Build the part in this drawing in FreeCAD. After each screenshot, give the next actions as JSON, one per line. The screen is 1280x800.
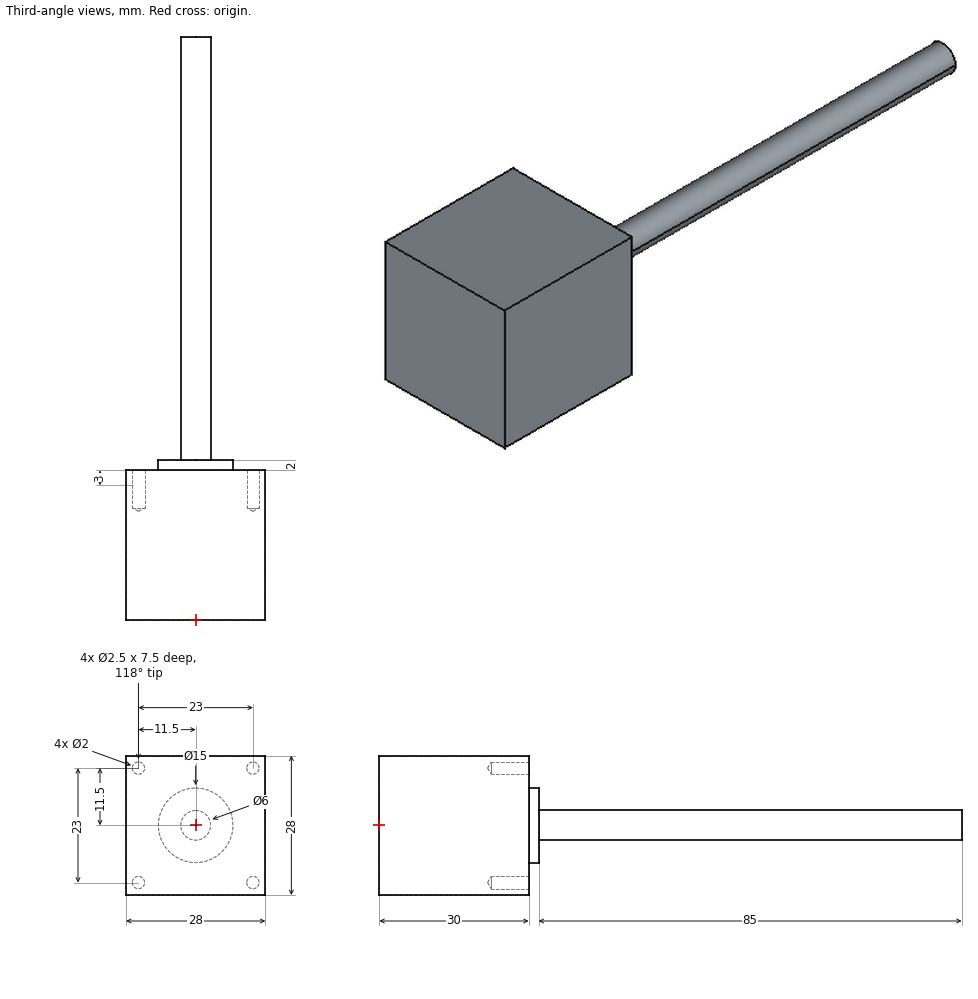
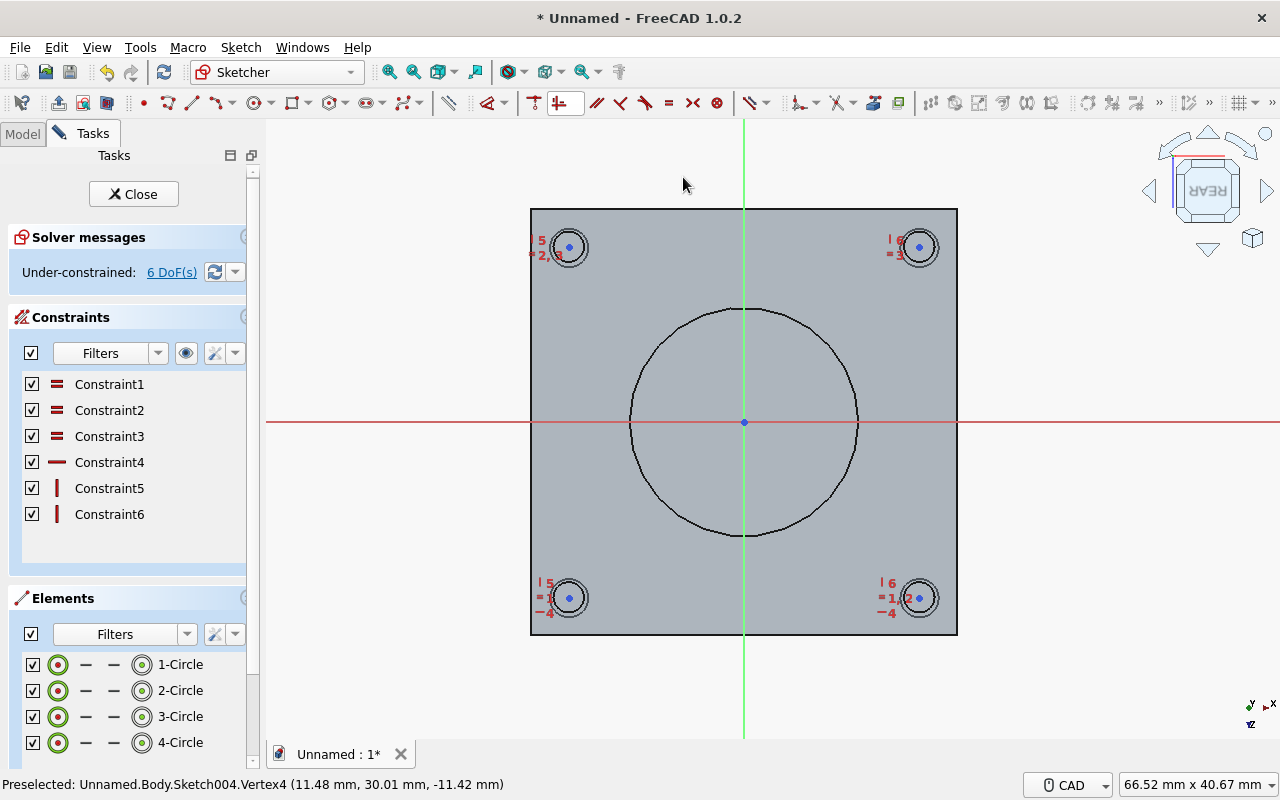
{"action": "left_click", "coordinate": [569, 248]}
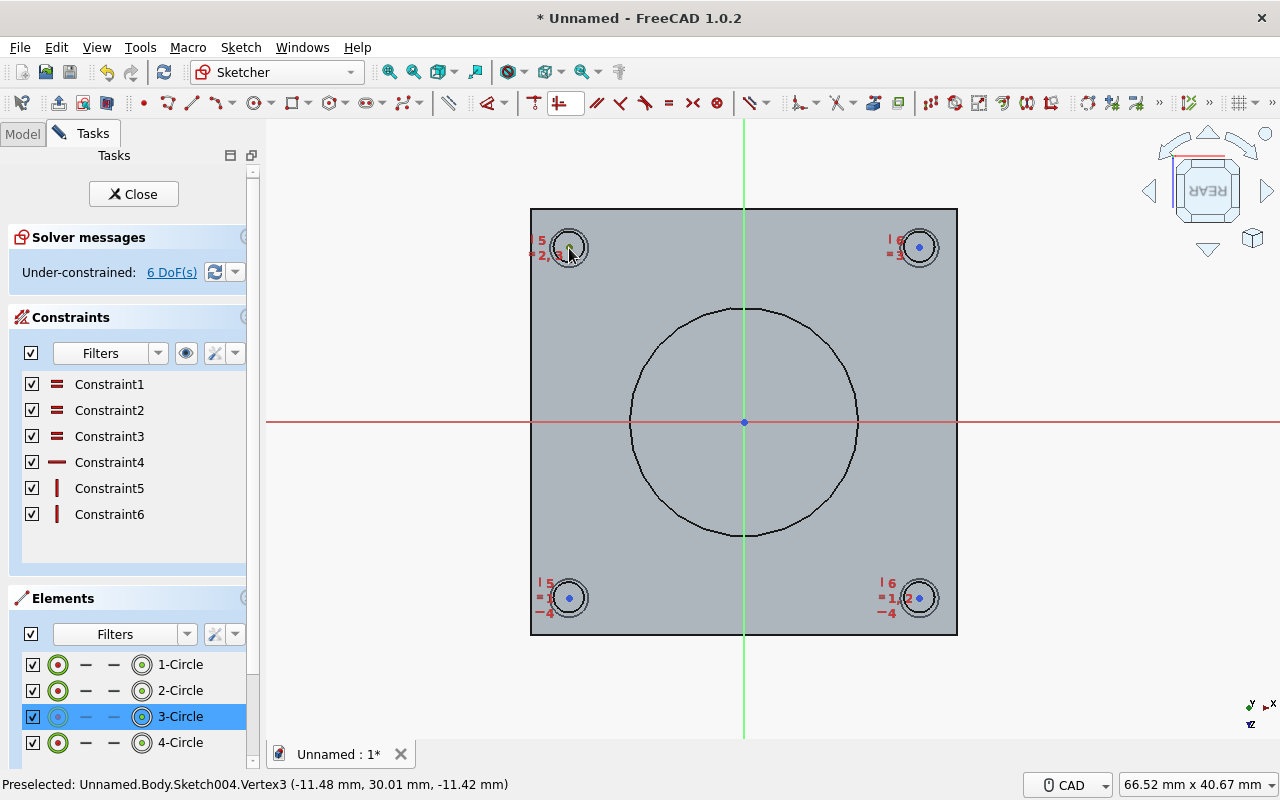
{"action": "left_click", "coordinate": [920, 248]}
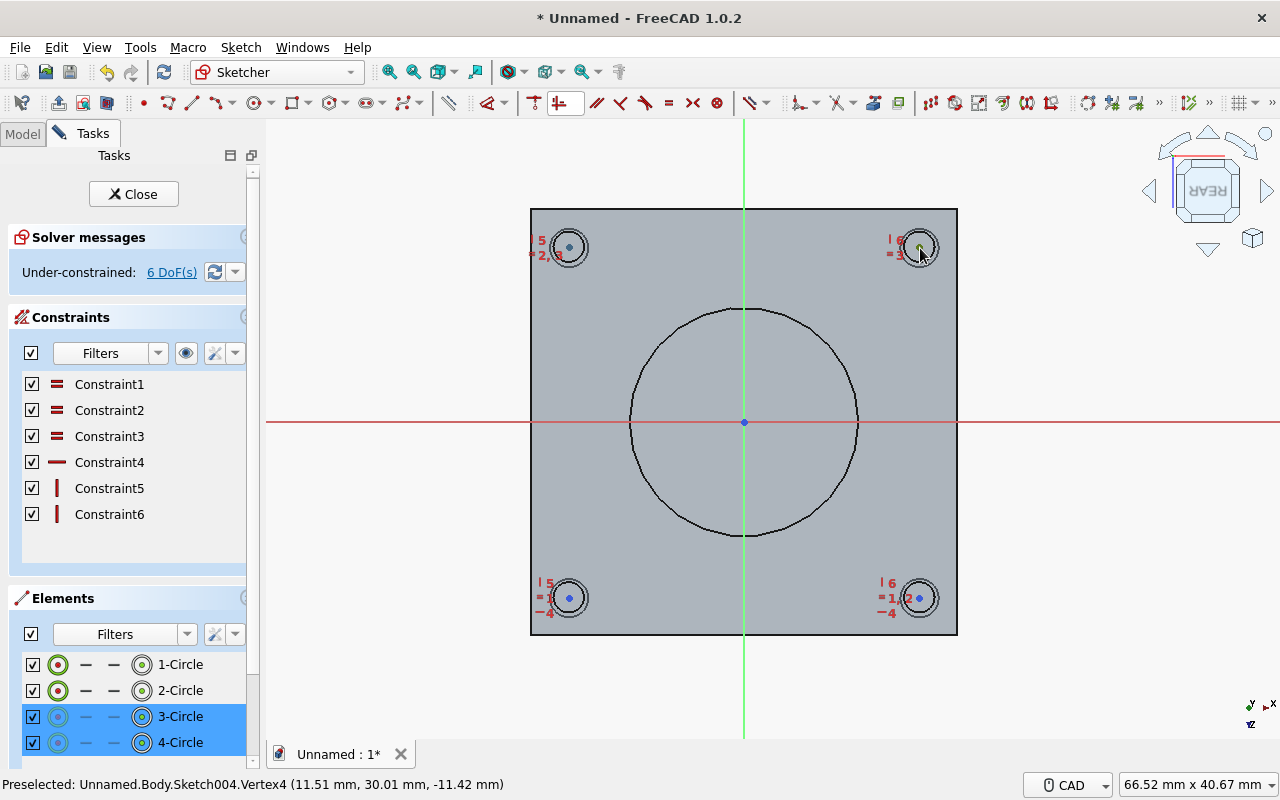
{"action": "left_click", "coordinate": [578, 104]}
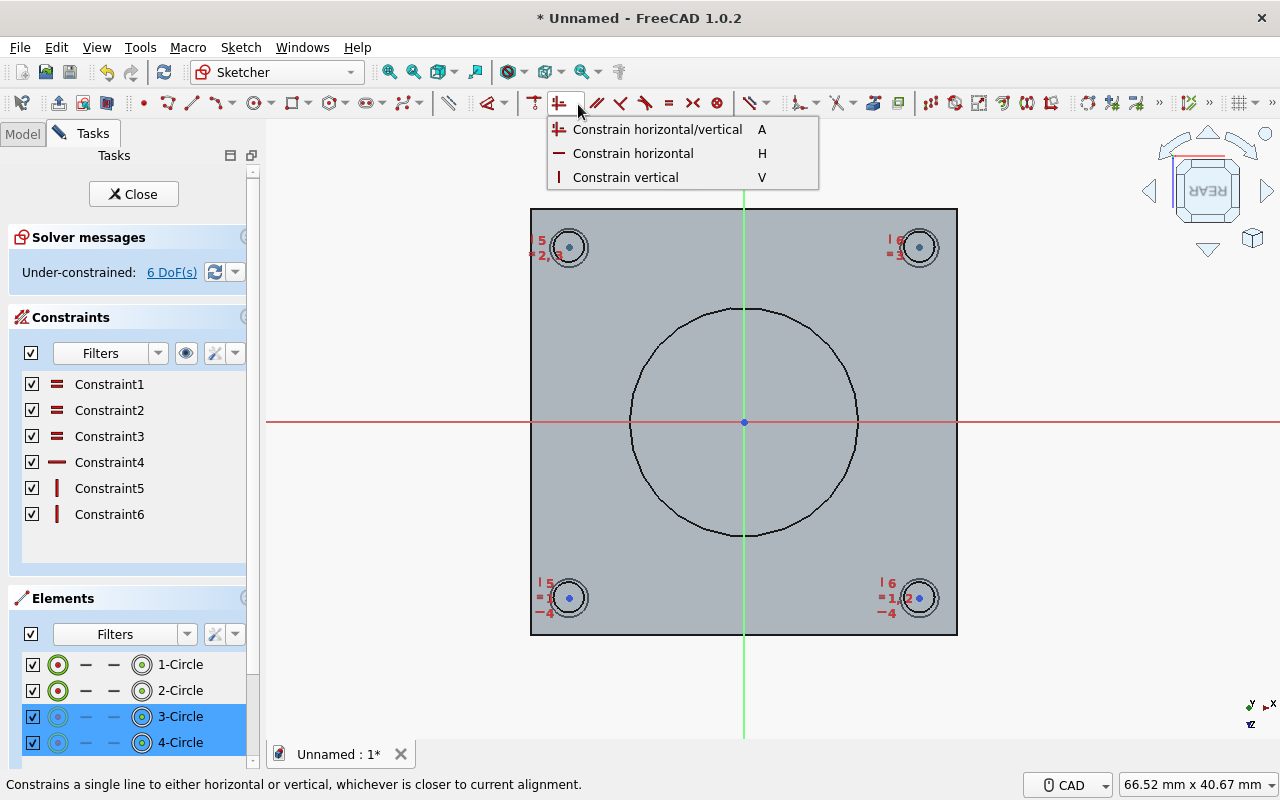
{"action": "left_click", "coordinate": [683, 153]}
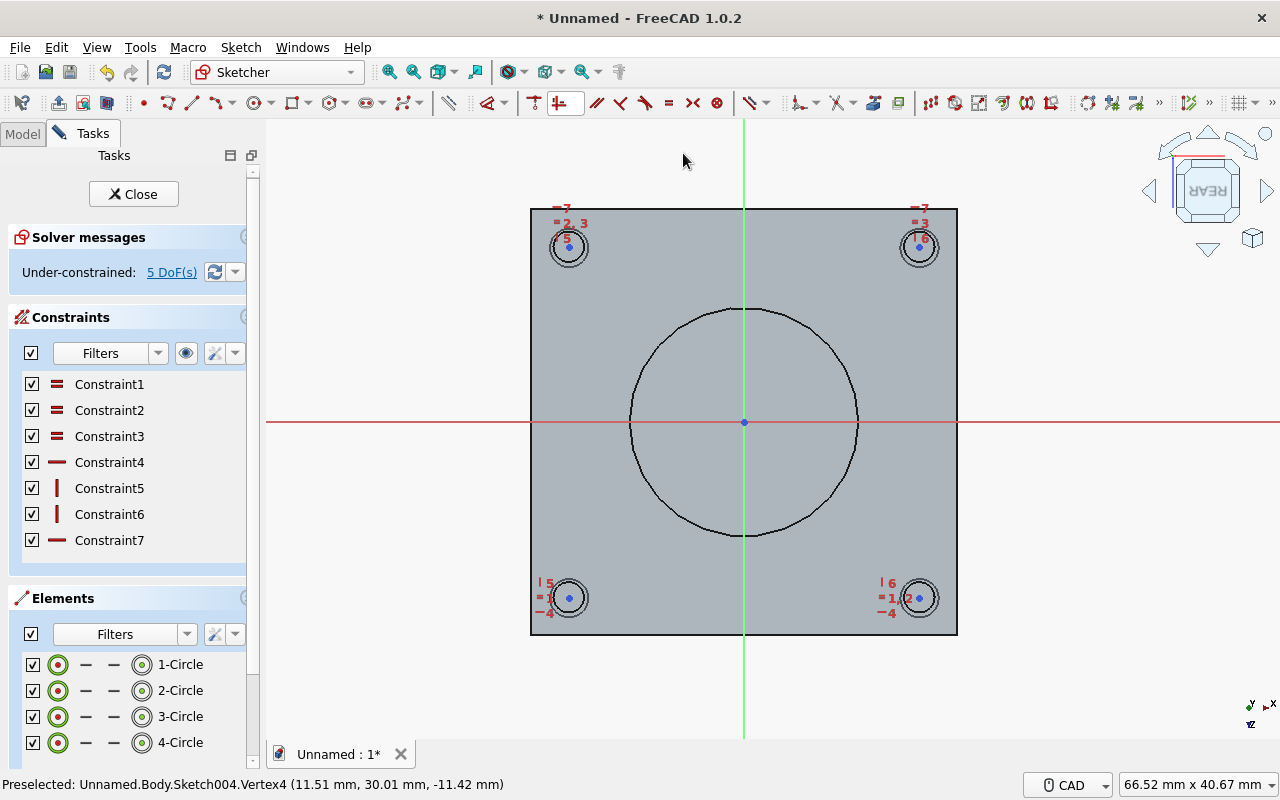
{"action": "left_click", "coordinate": [488, 104]}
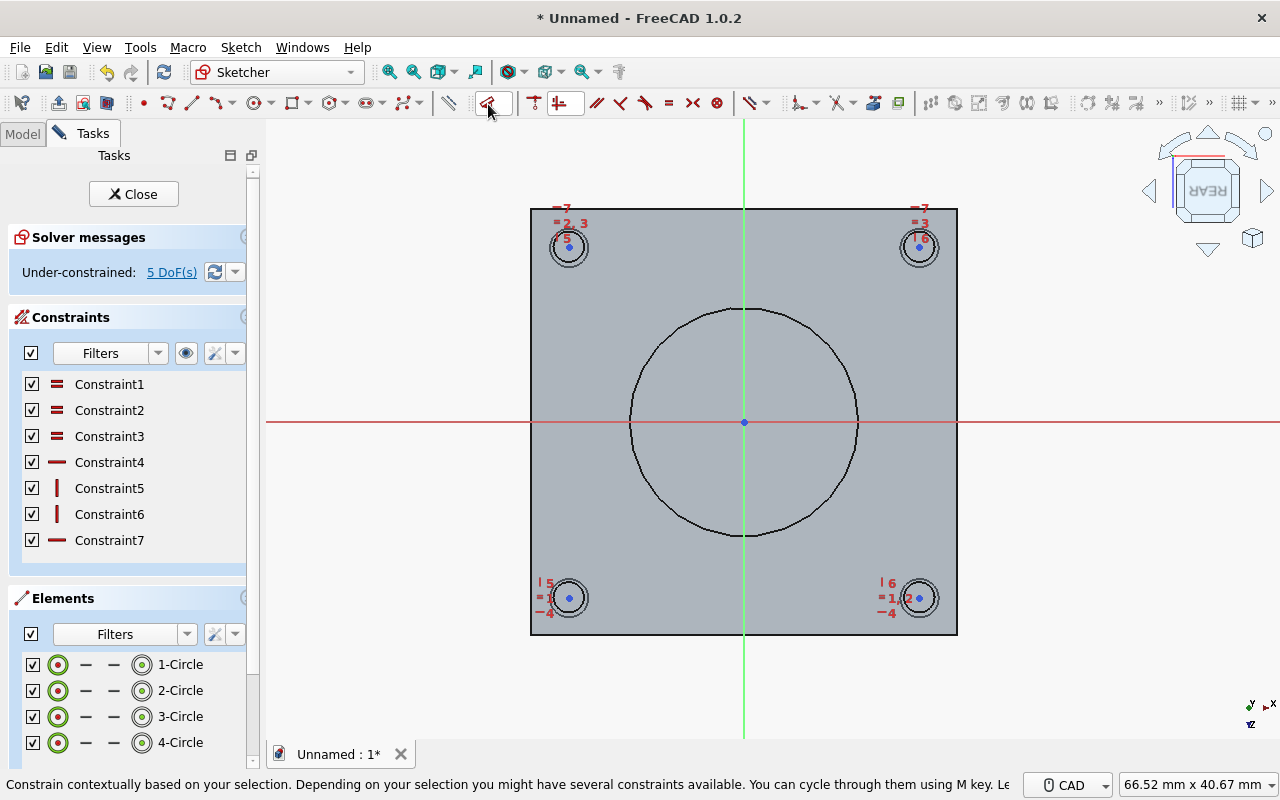
{"action": "left_click", "coordinate": [583, 585]}
{"action": "left_click", "coordinate": [606, 563]}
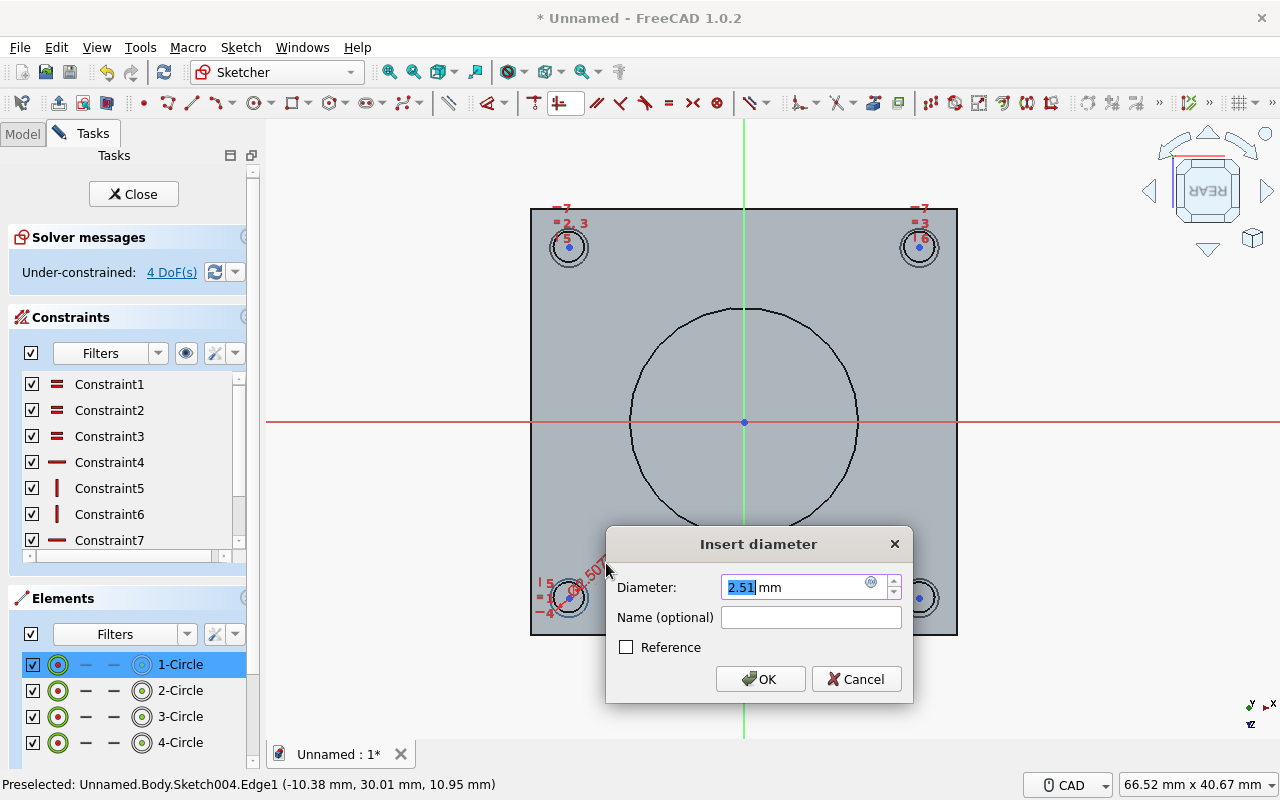
{"action": "type", "text": "2.5"}
{"action": "key", "text": "Return"}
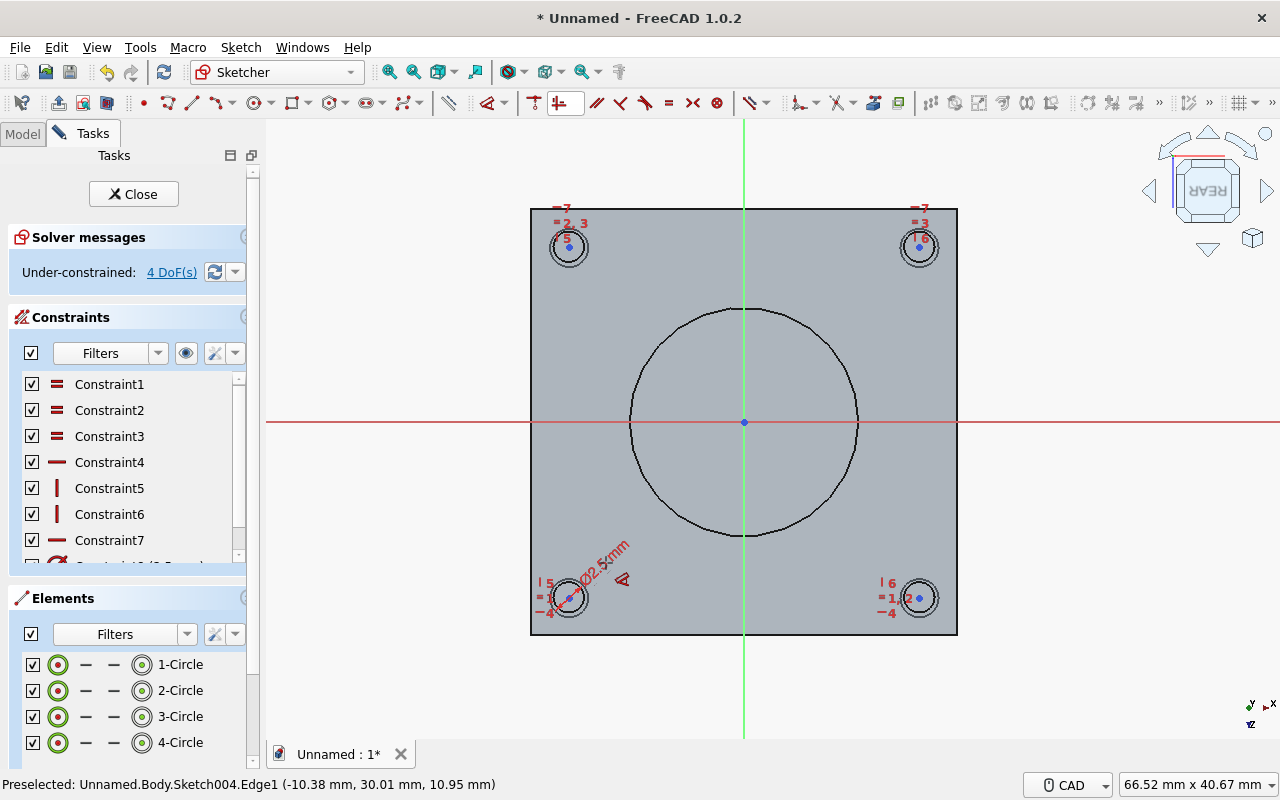
{"action": "left_click", "coordinate": [569, 598]}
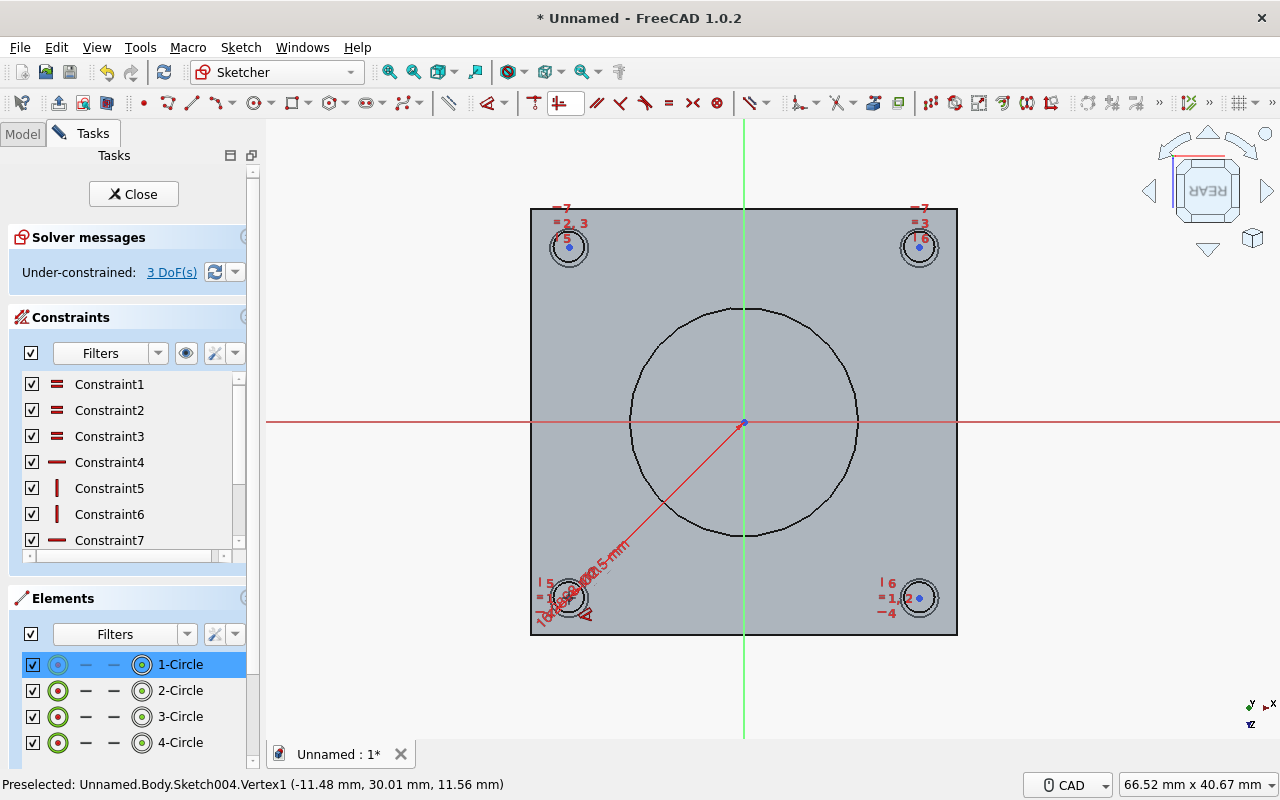
{"action": "left_click", "coordinate": [920, 598]}
{"action": "left_click", "coordinate": [664, 632]}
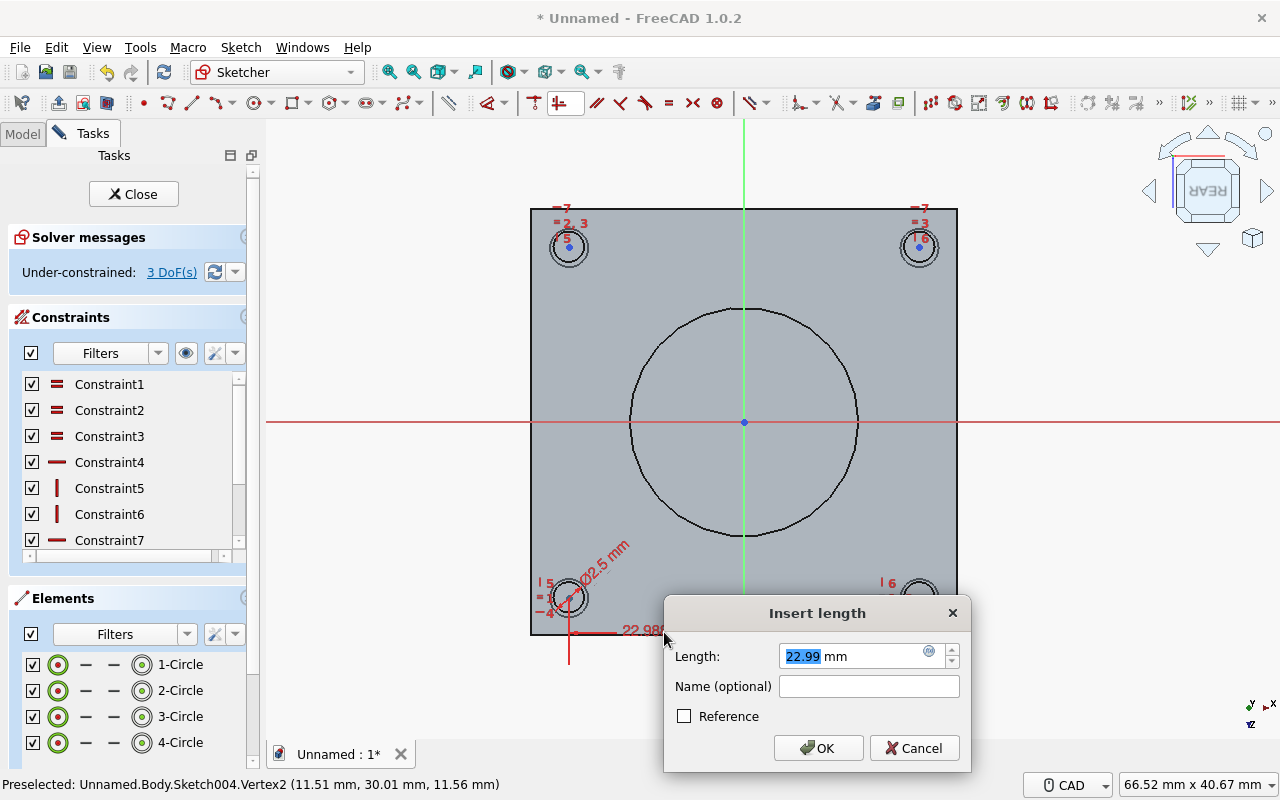
{"action": "type", "text": "23"}
{"action": "key", "text": "Return"}